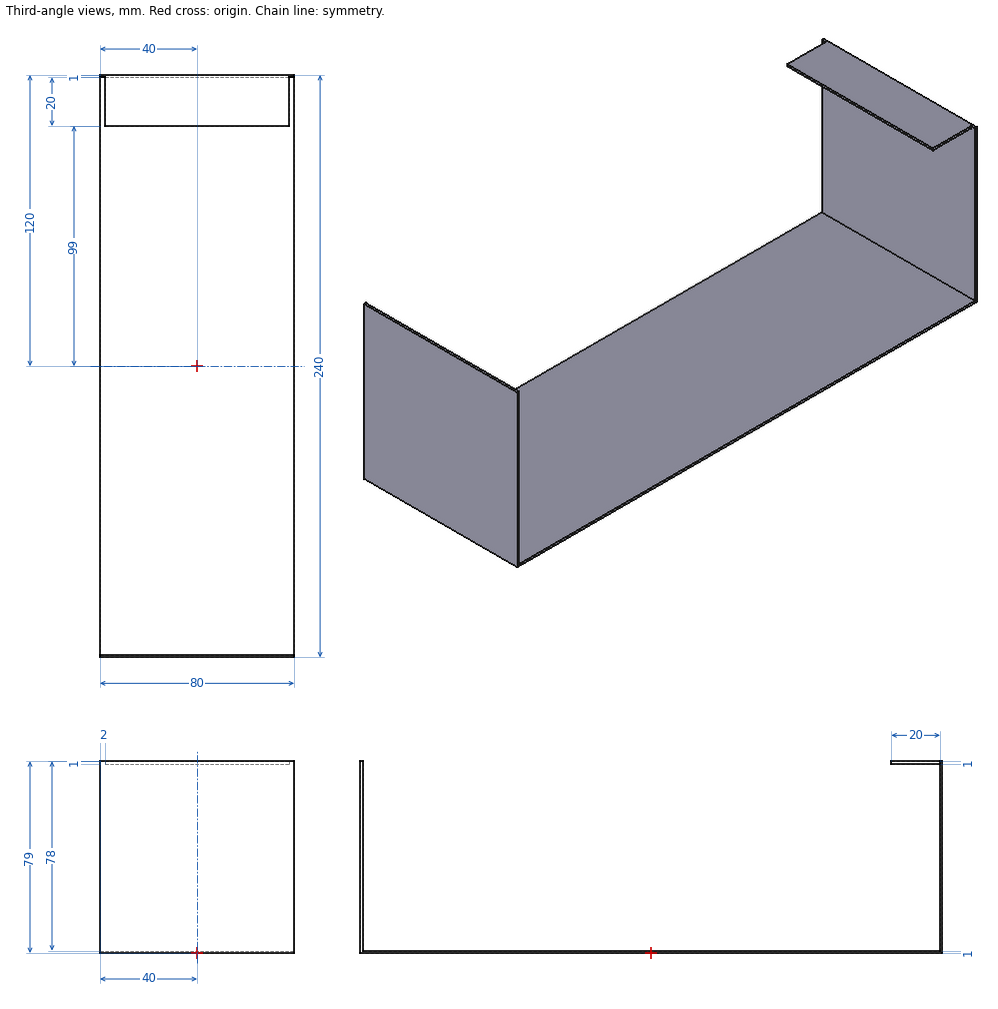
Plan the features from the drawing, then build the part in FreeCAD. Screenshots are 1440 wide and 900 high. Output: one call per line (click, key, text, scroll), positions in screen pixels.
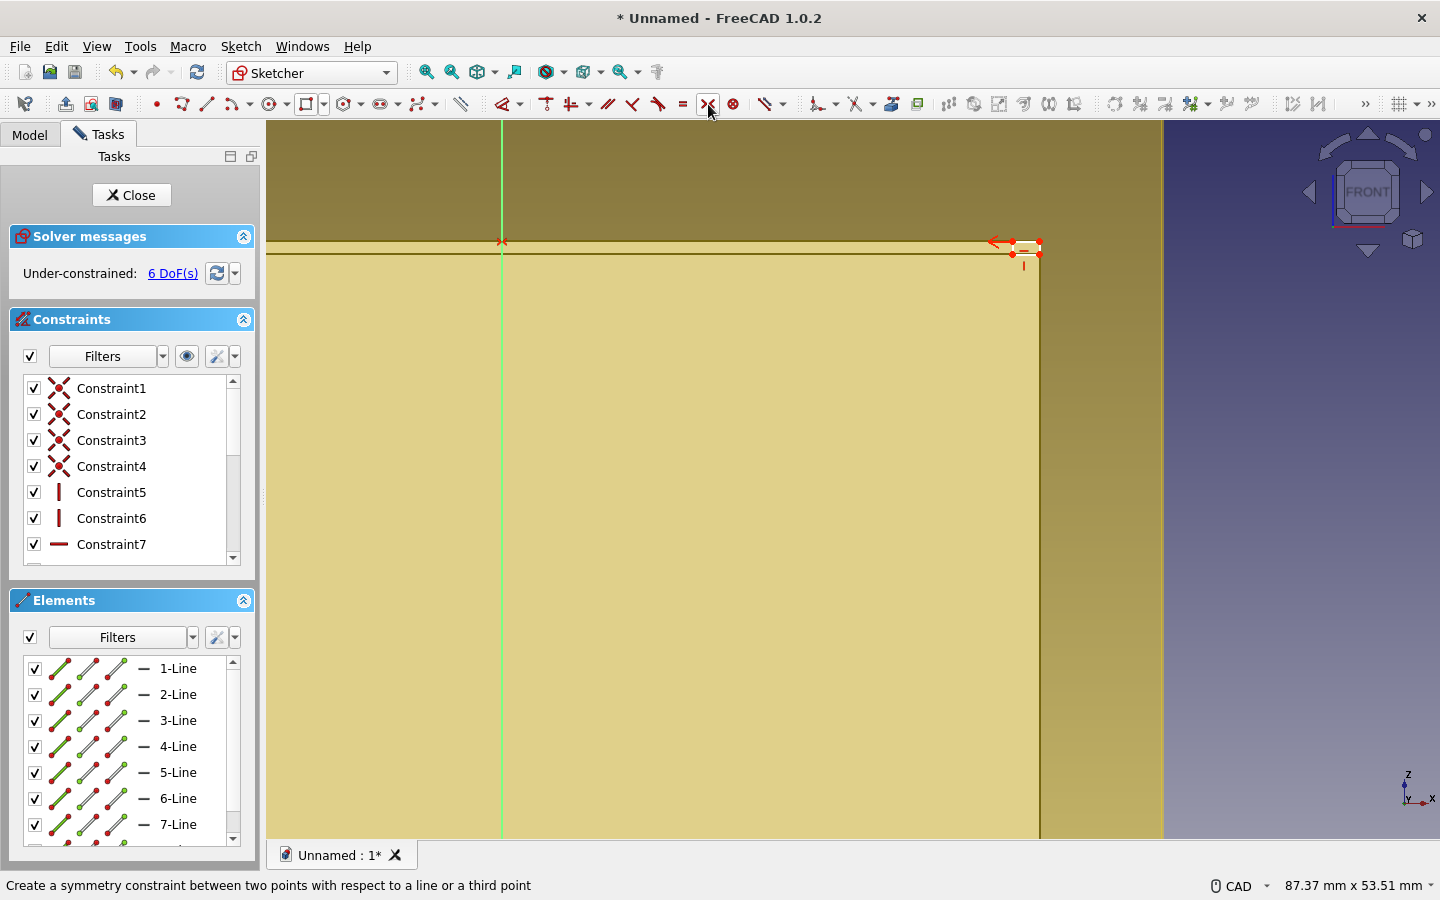
scroll(1015, 241, down, 4)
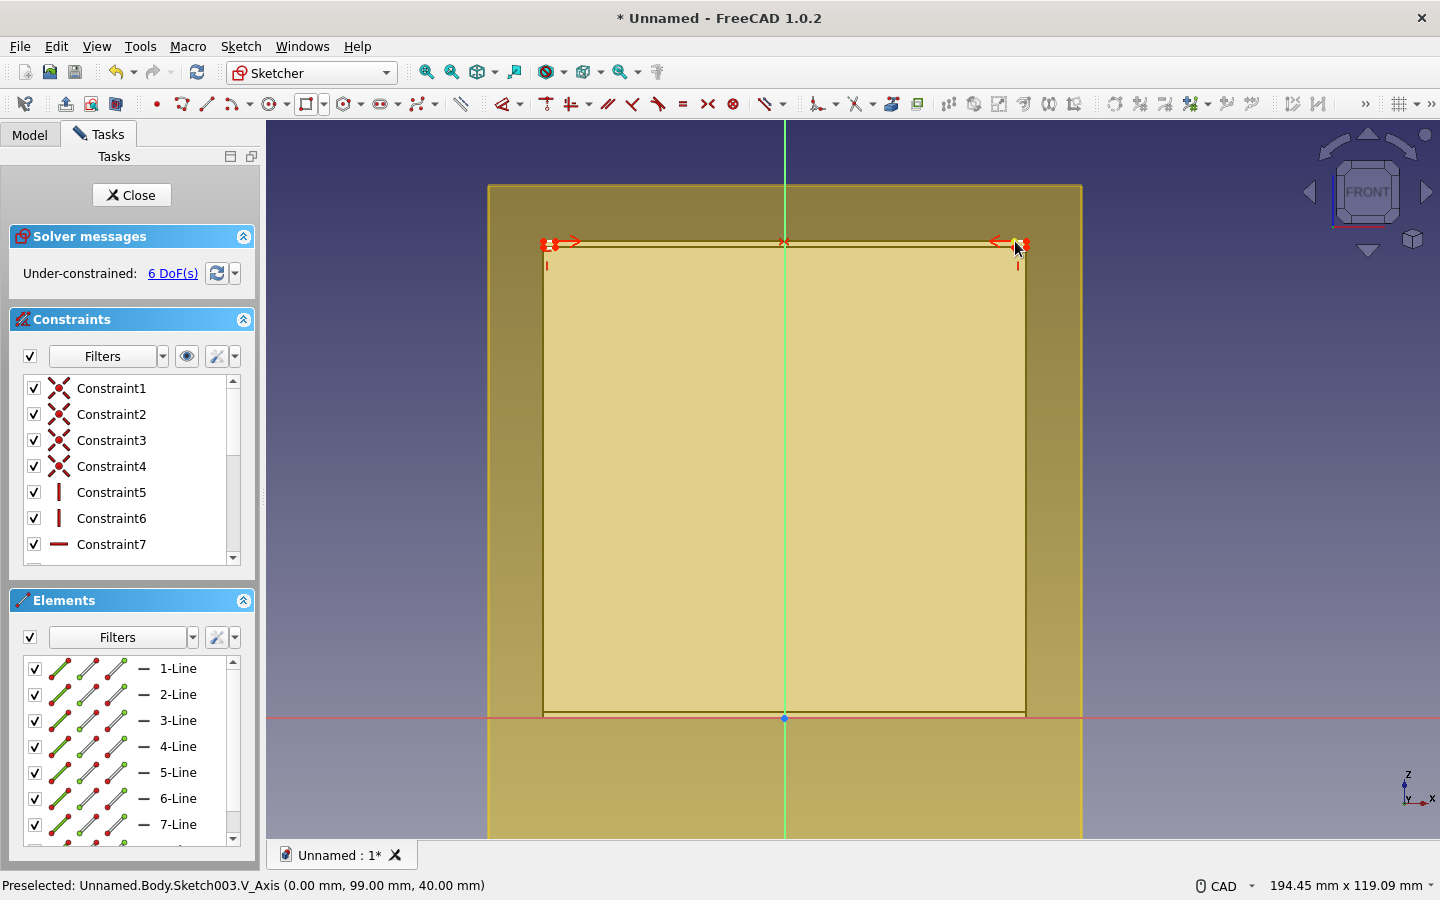
scroll(543, 248, up, 4)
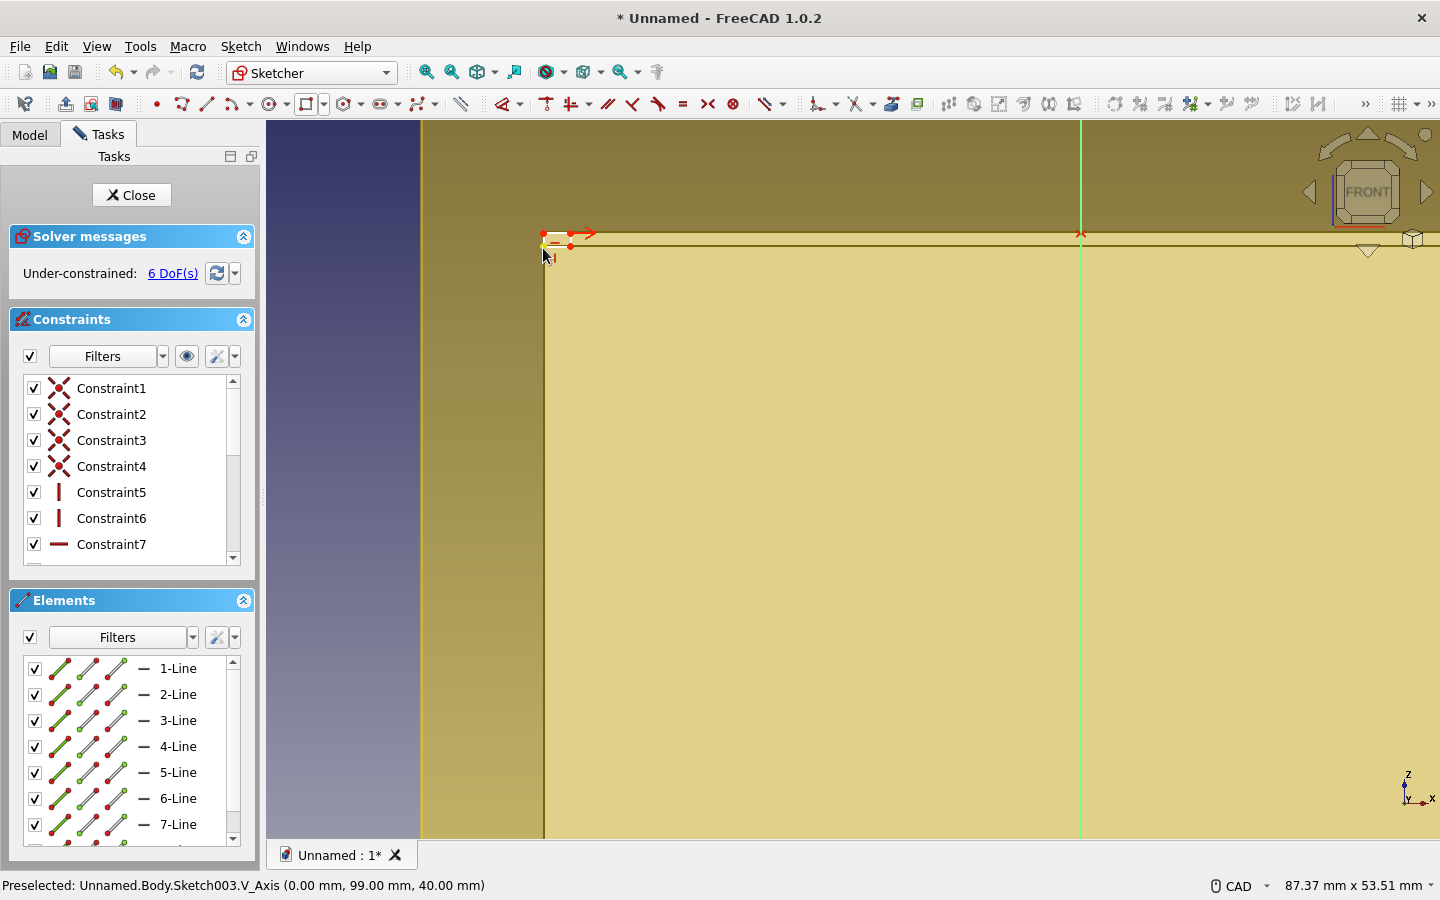
click(544, 247)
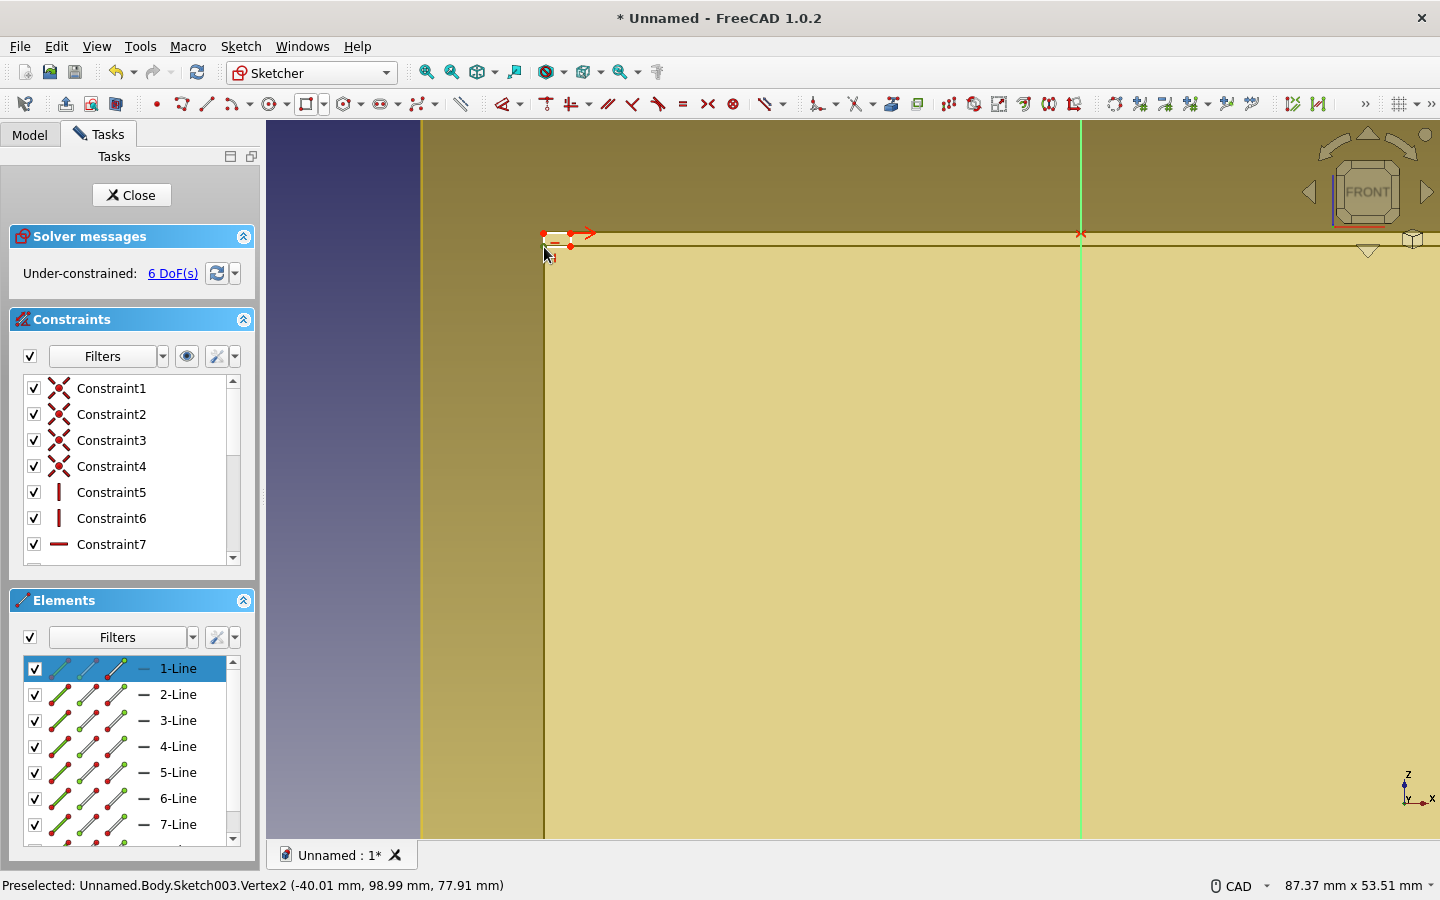
scroll(542, 248, down, 4)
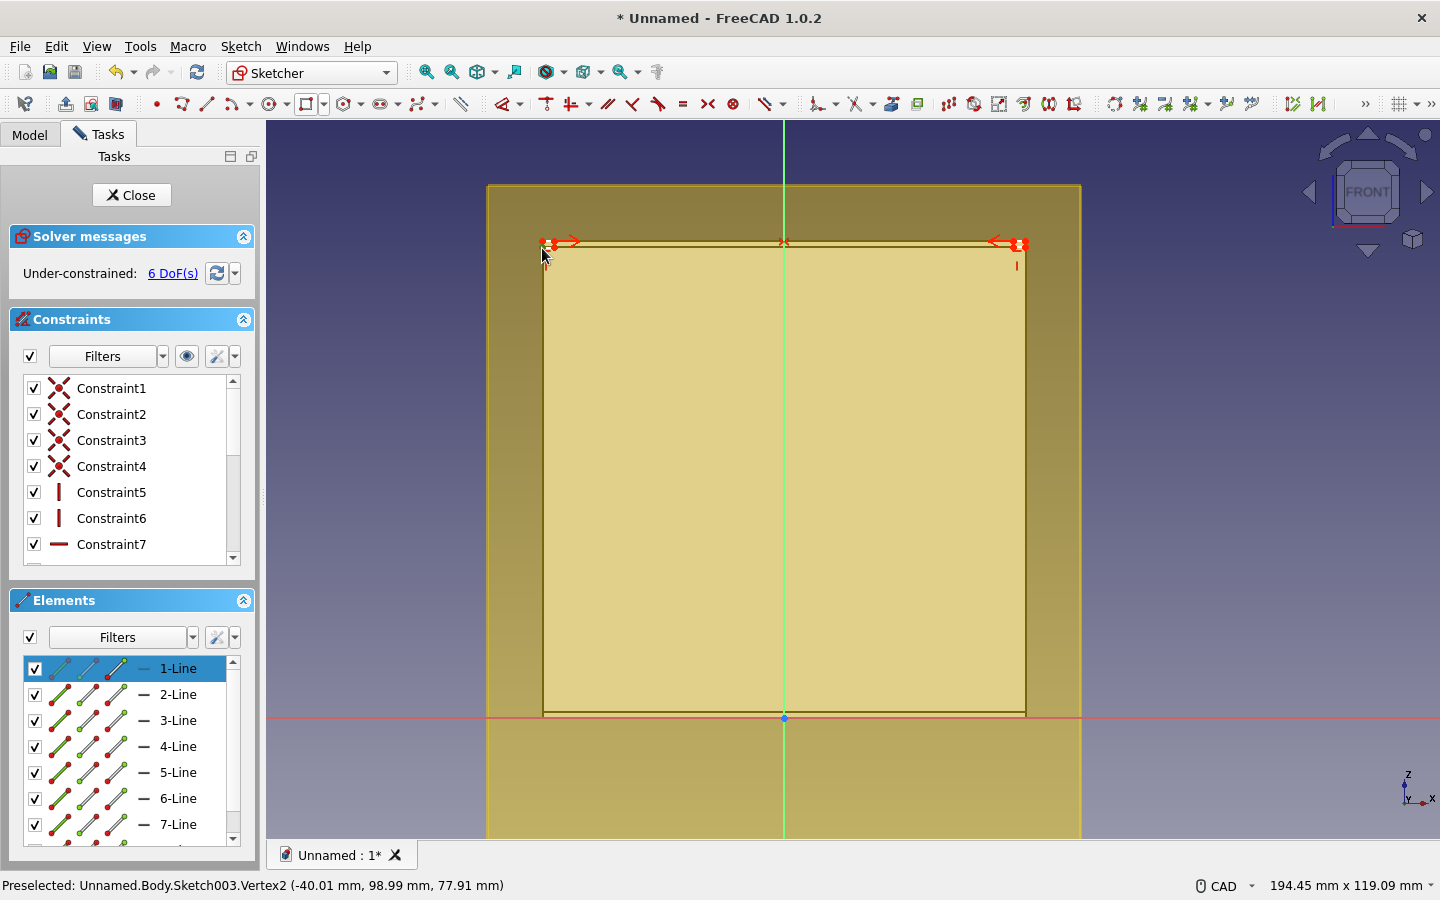
scroll(1026, 247, up, 4)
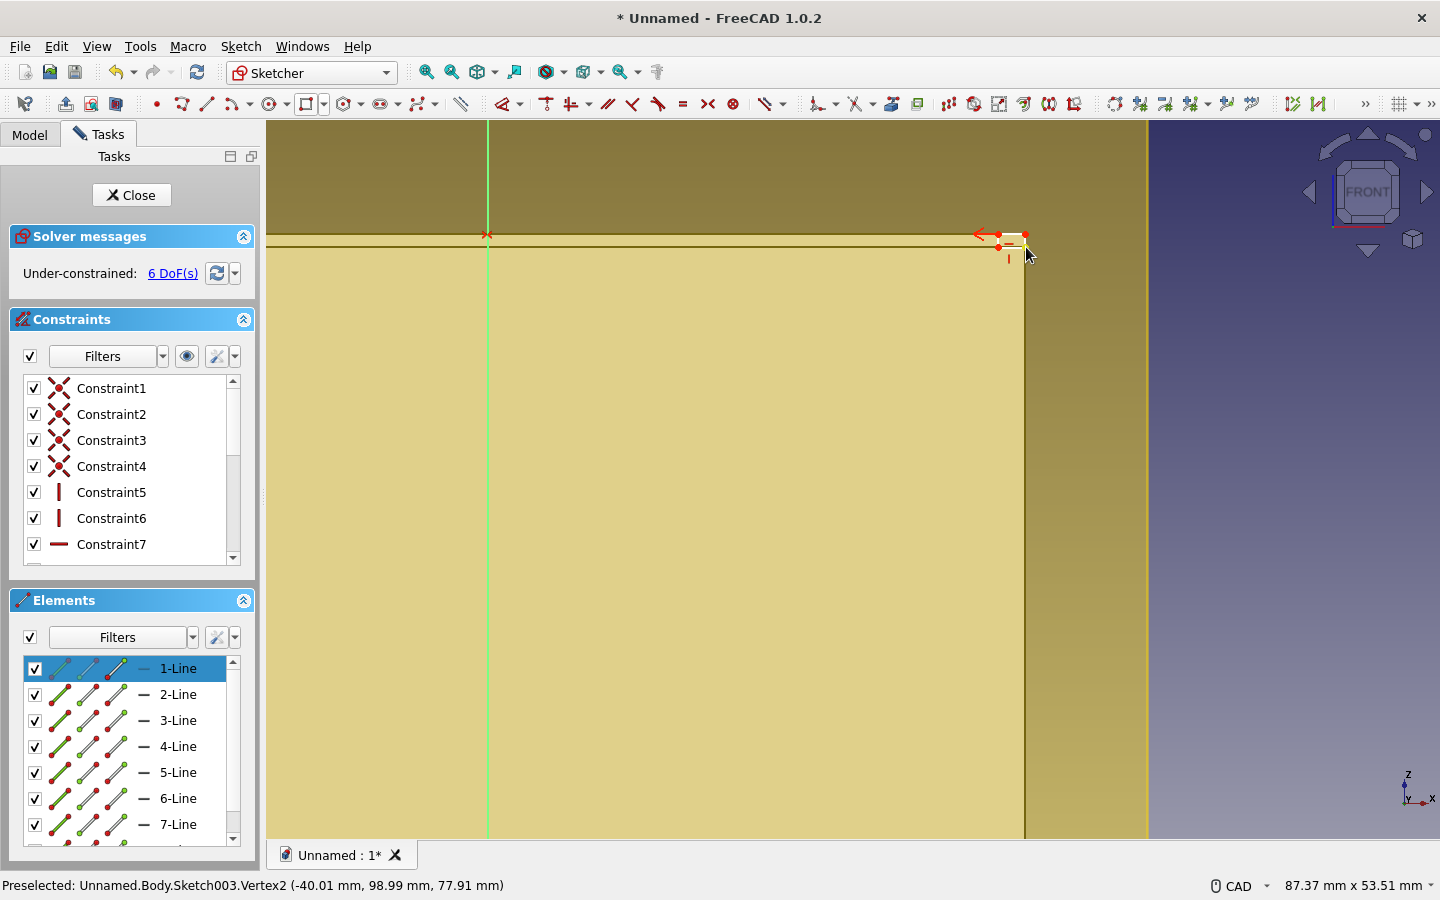
click(1025, 248)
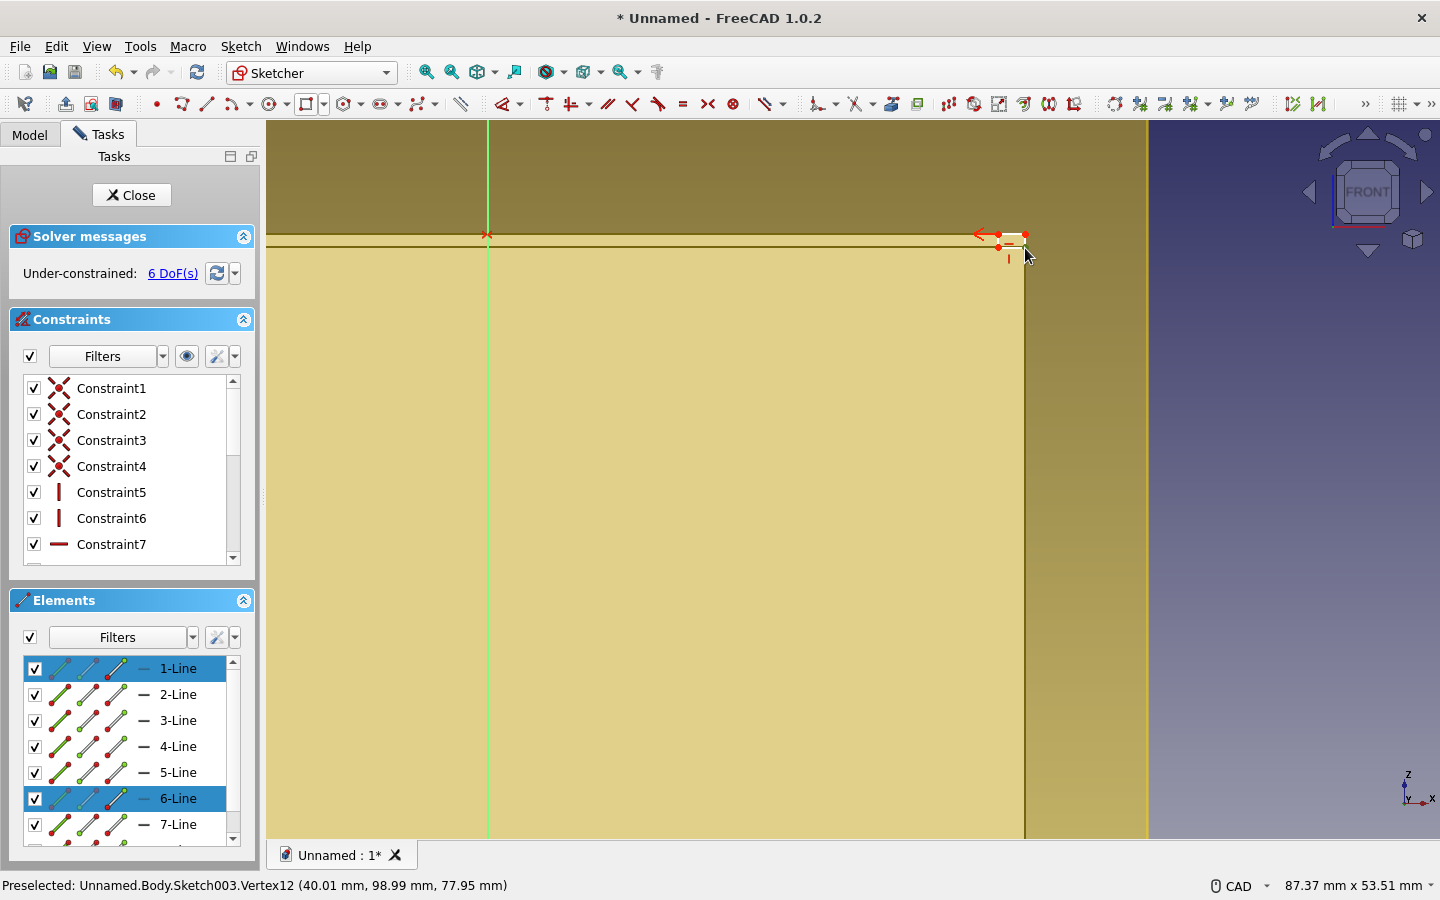
click(488, 764)